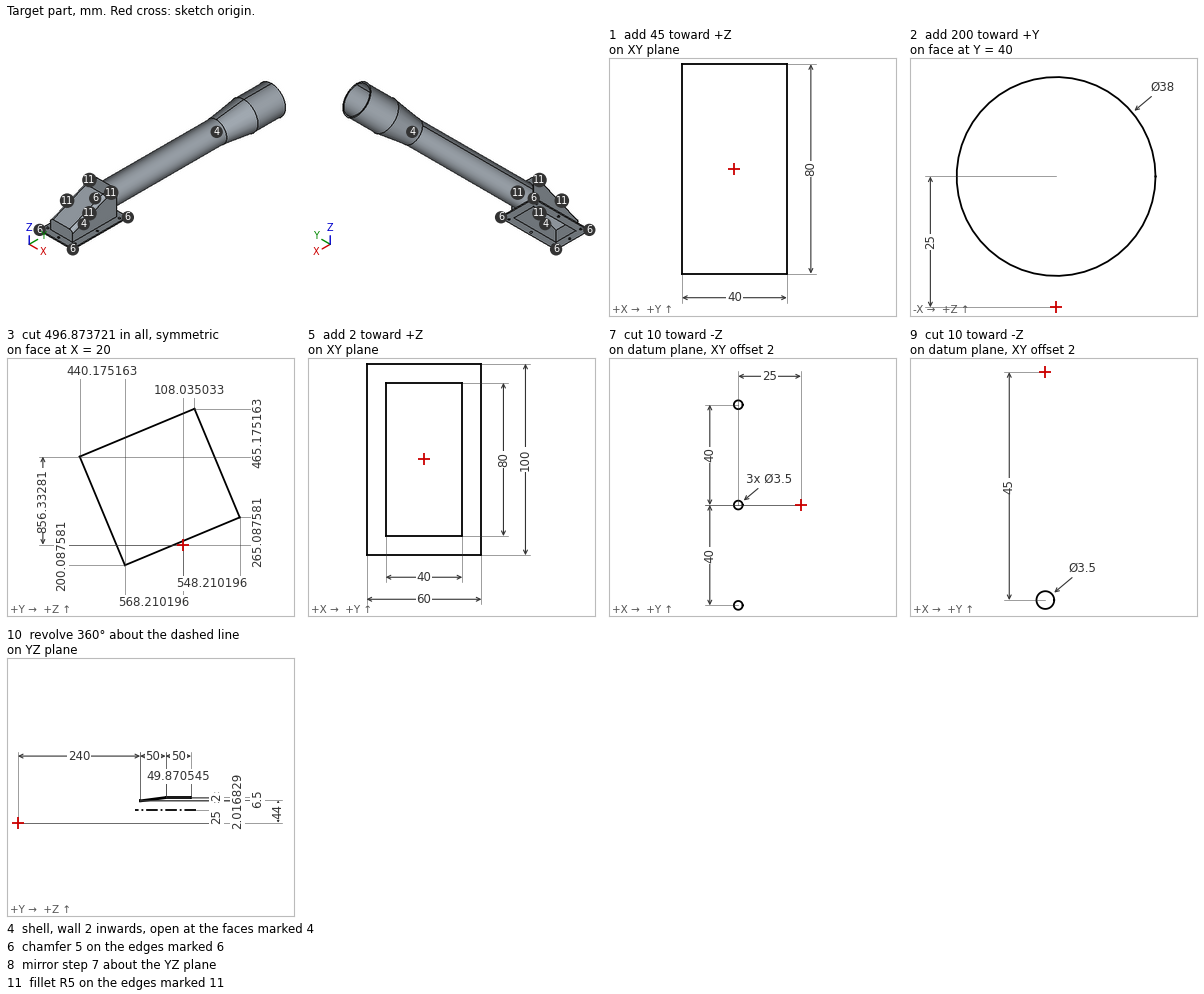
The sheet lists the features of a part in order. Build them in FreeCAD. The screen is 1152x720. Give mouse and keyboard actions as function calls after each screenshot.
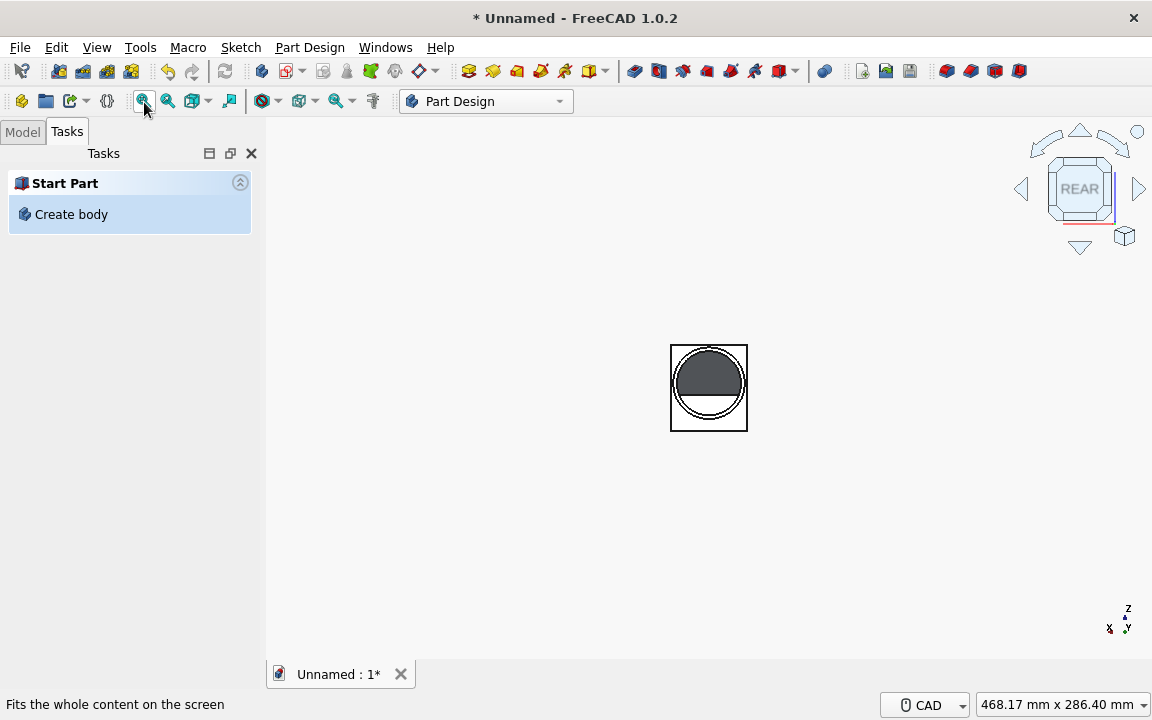
click(286, 72)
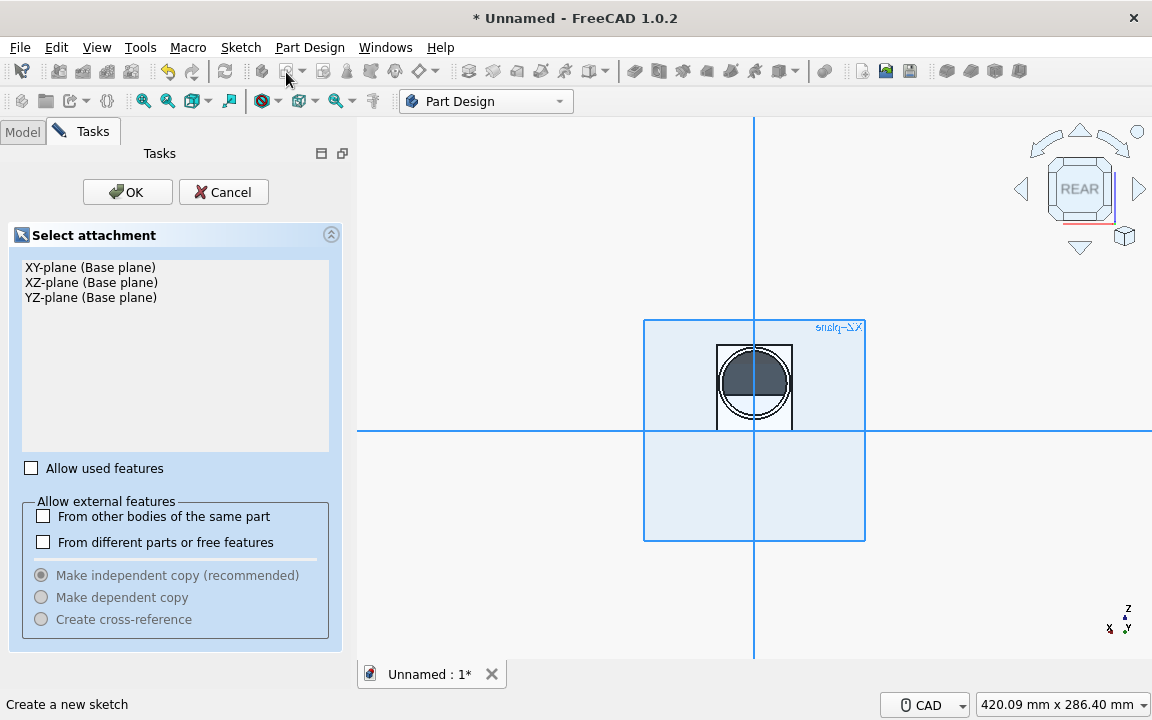
click(82, 268)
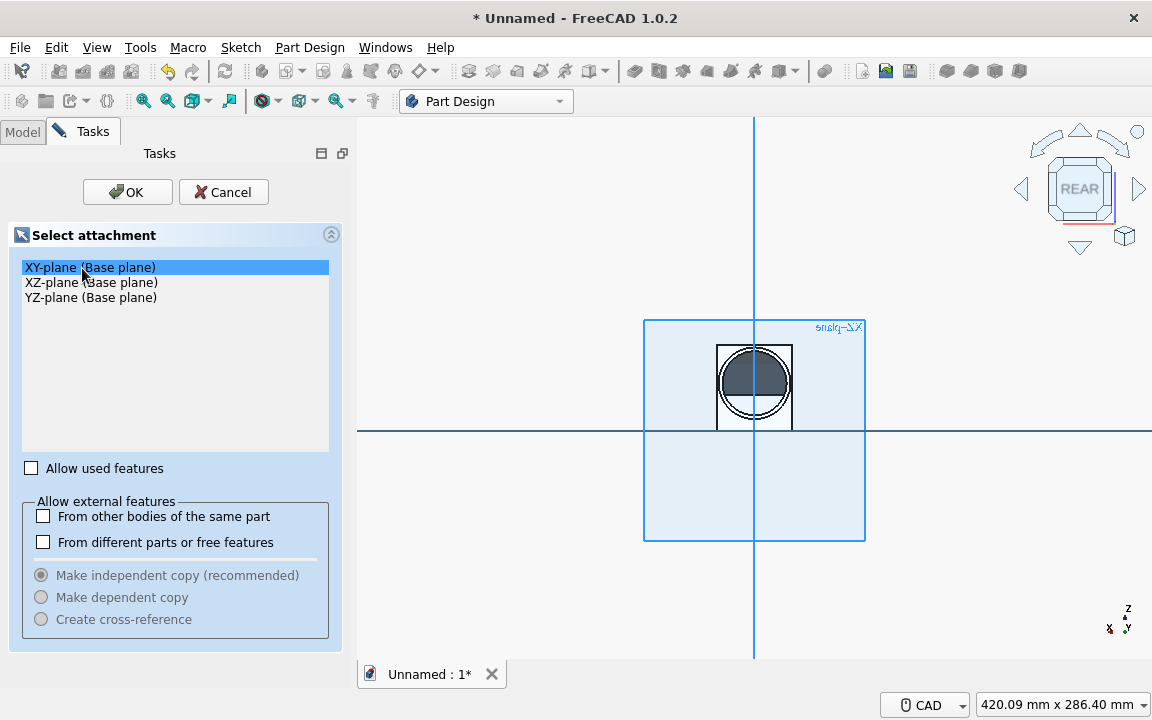
click(128, 192)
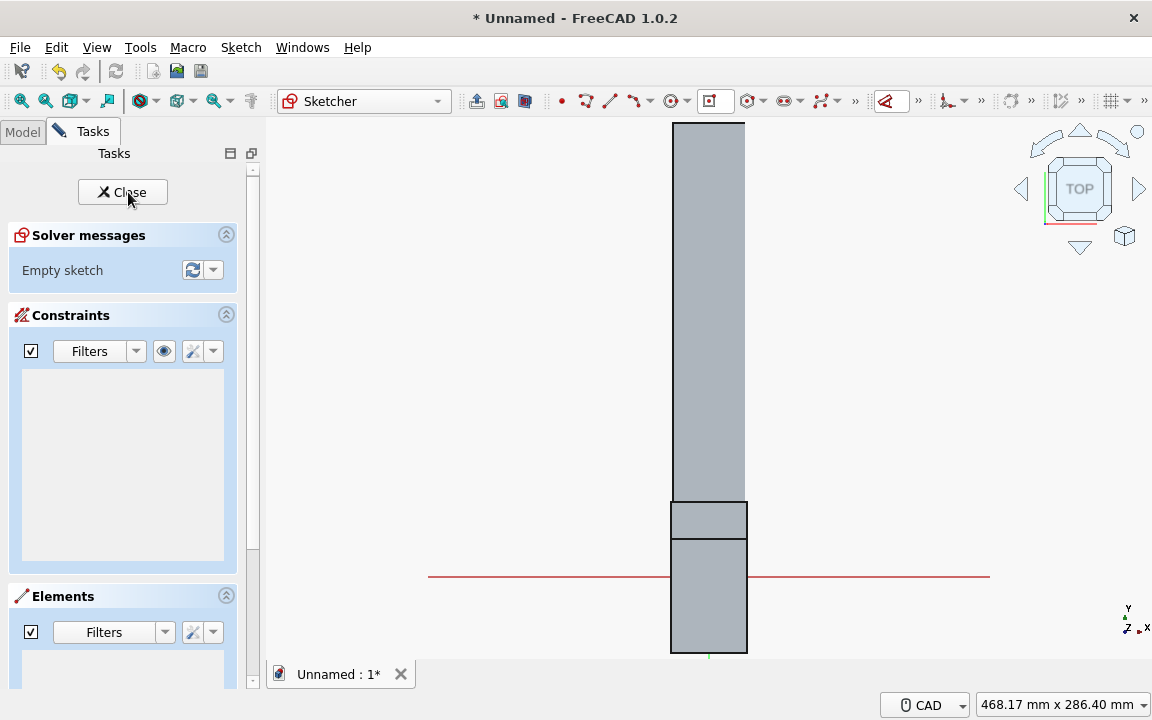
key(q)
key(s)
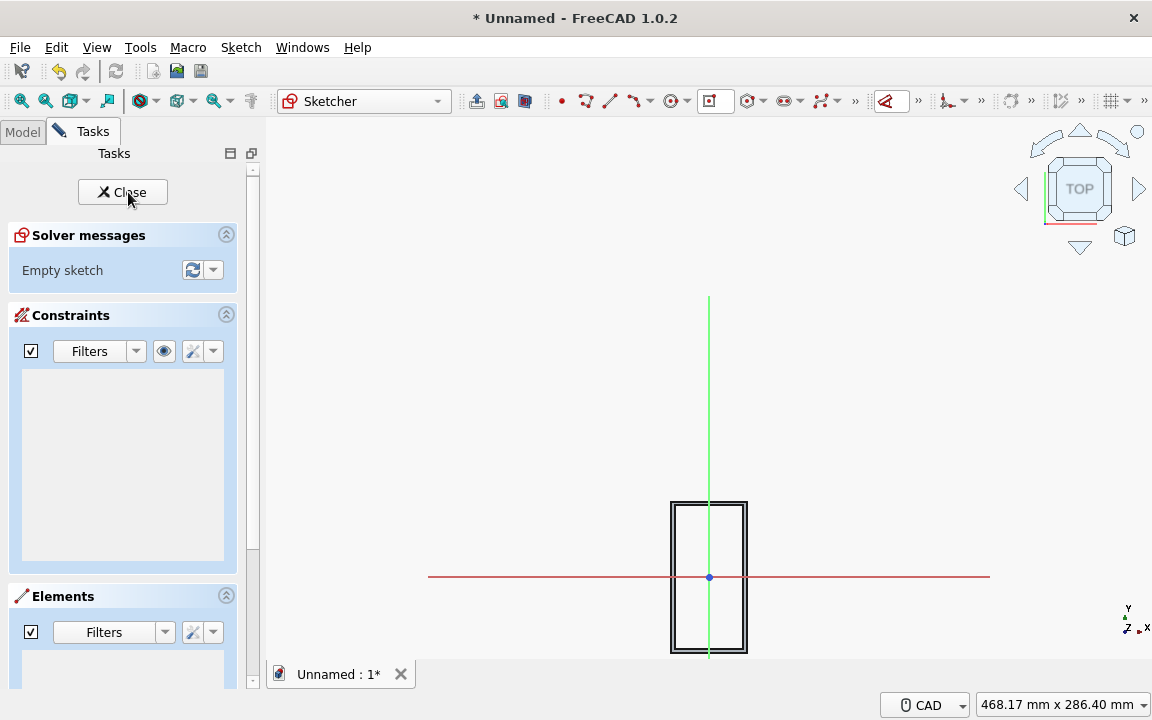
scroll(640, 388, down, 5)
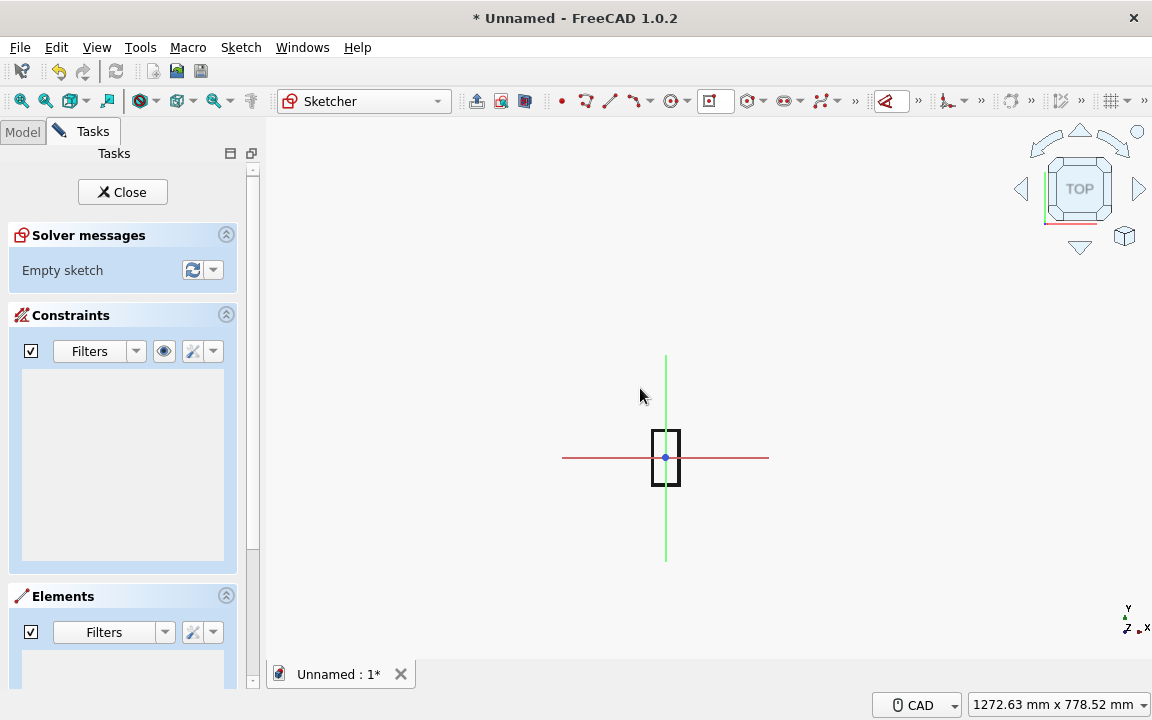
scroll(672, 476, up, 8)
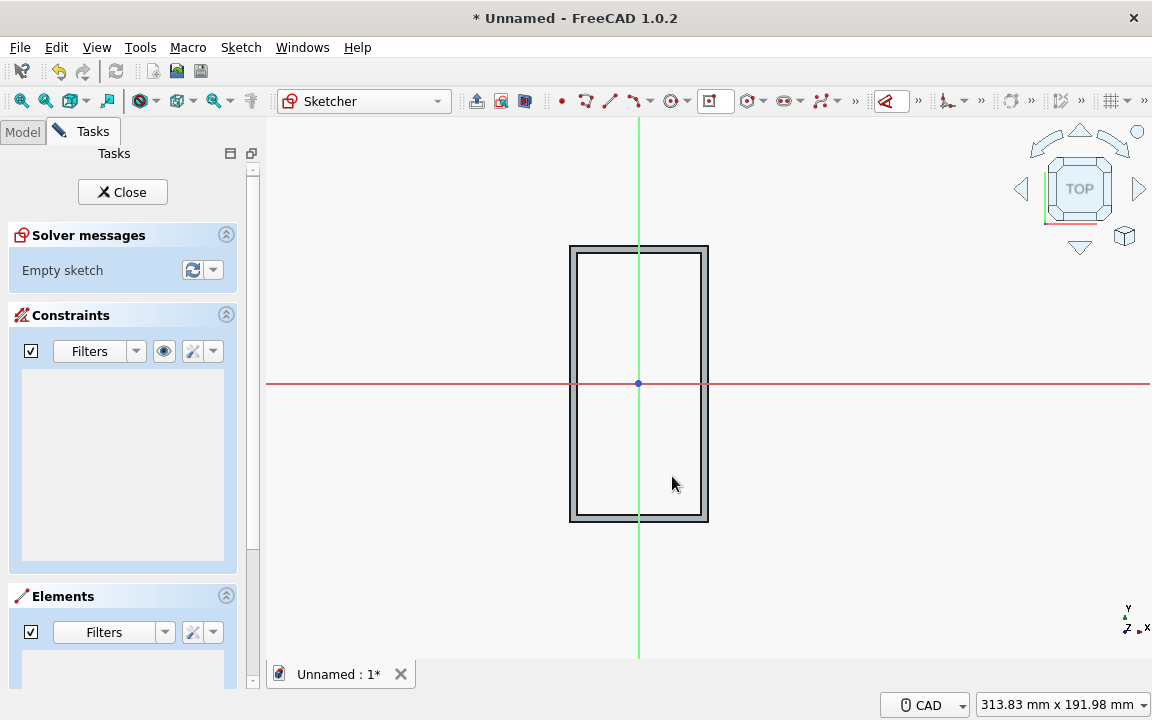
key(g)
key(v)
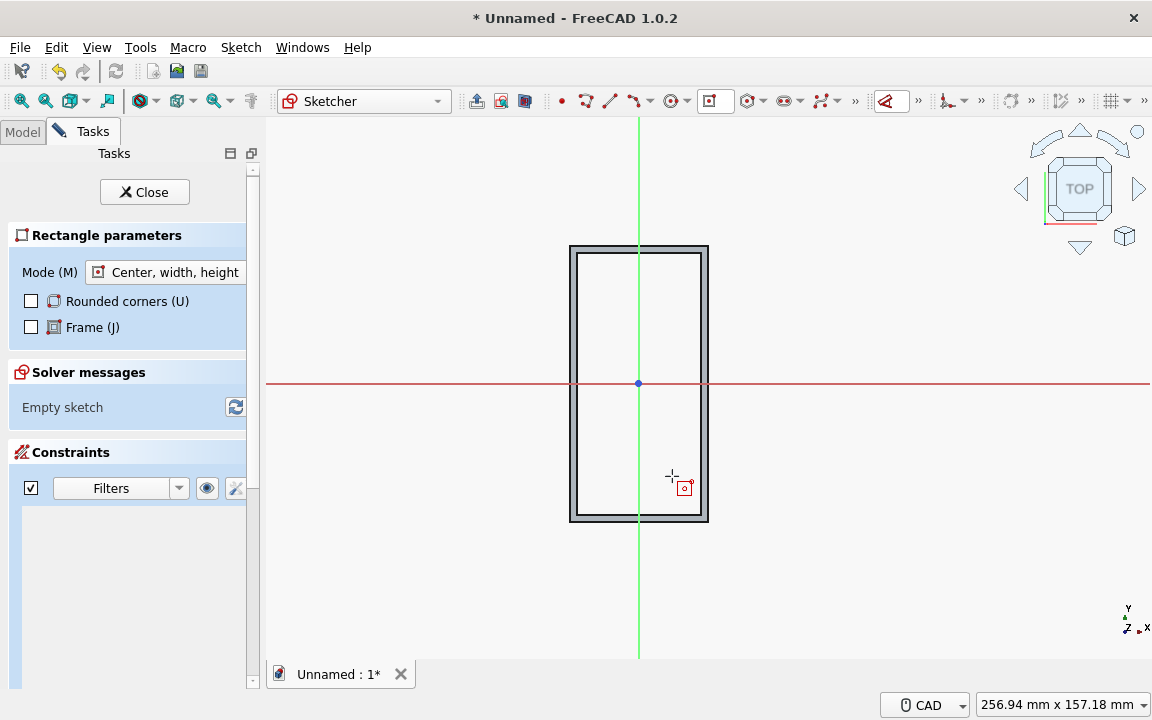
click(639, 384)
move(742, 211)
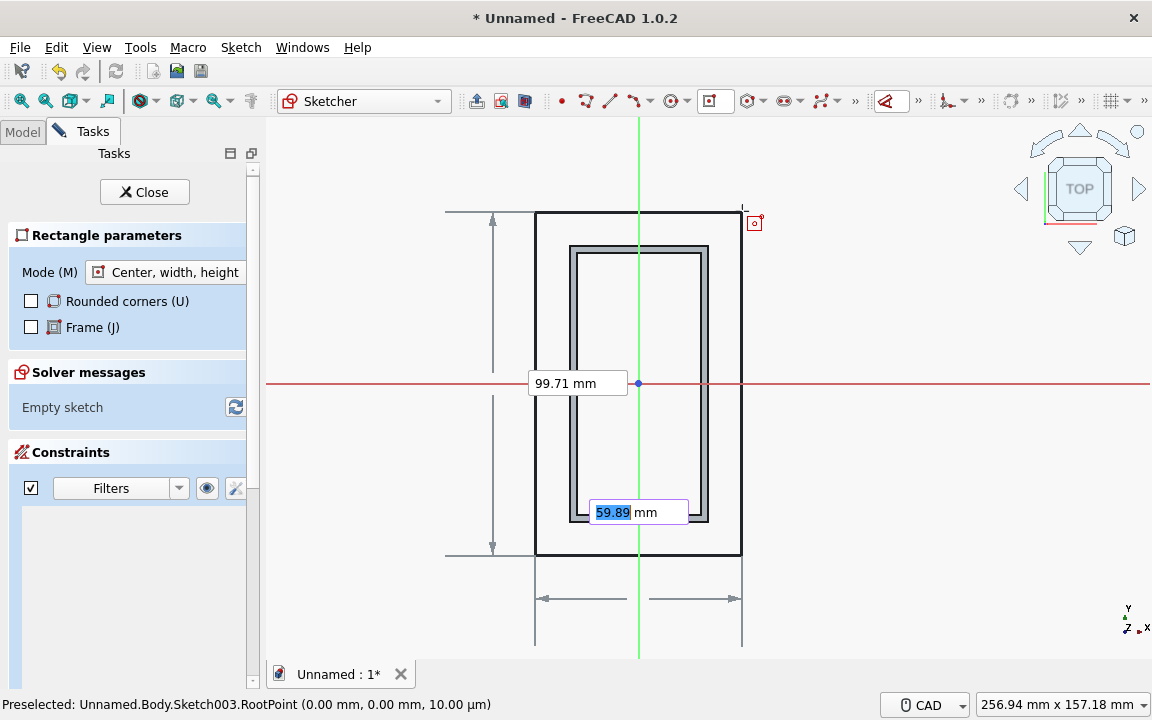
text(60)
key(Tab)
text(100)
key(Return)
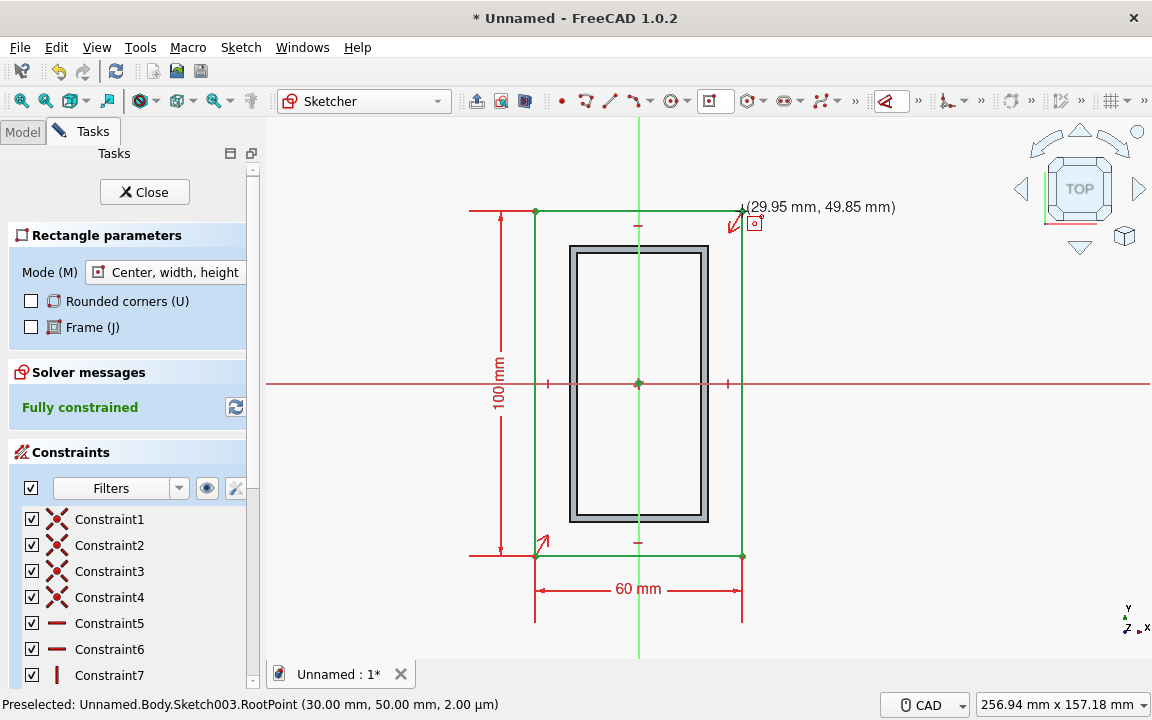
click(639, 384)
move(708, 246)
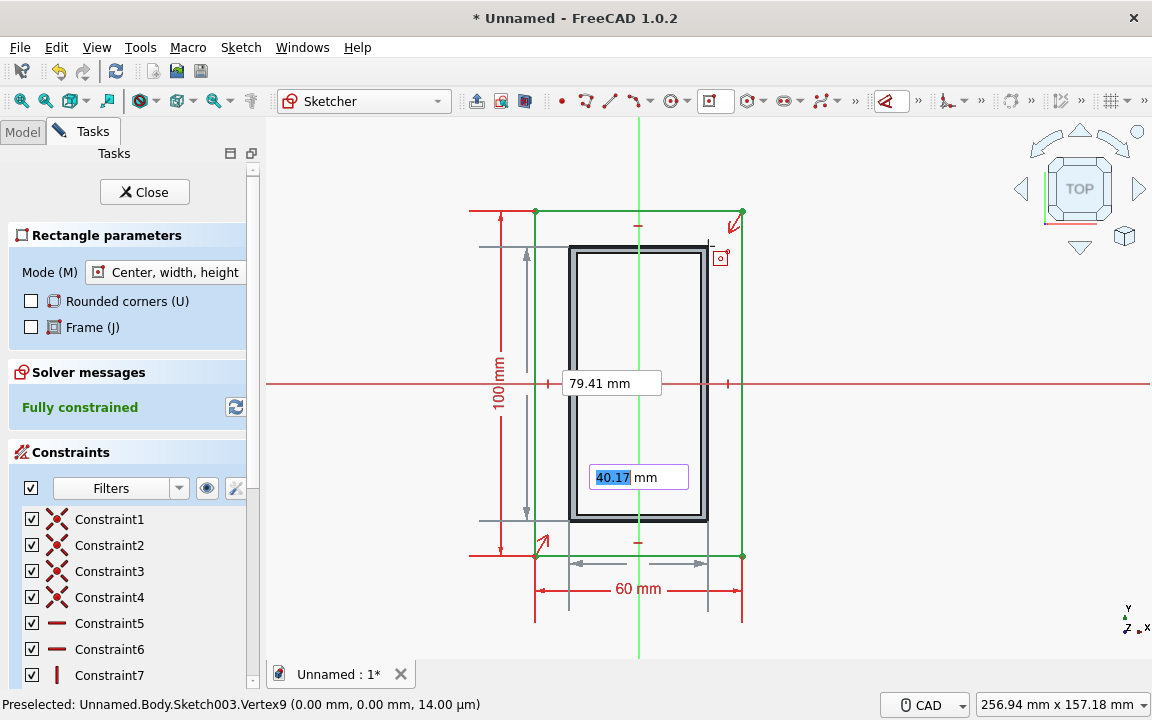
text(40)
key(Tab)
text(80)
key(Return)
key(Escape)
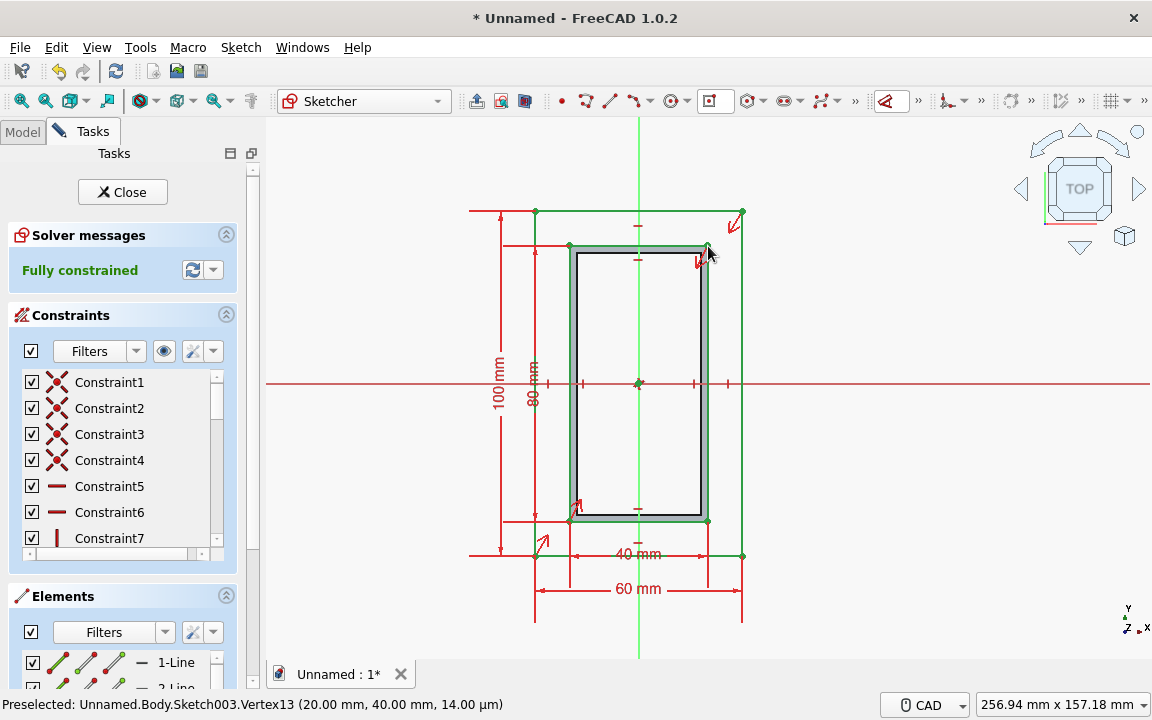
click(123, 192)